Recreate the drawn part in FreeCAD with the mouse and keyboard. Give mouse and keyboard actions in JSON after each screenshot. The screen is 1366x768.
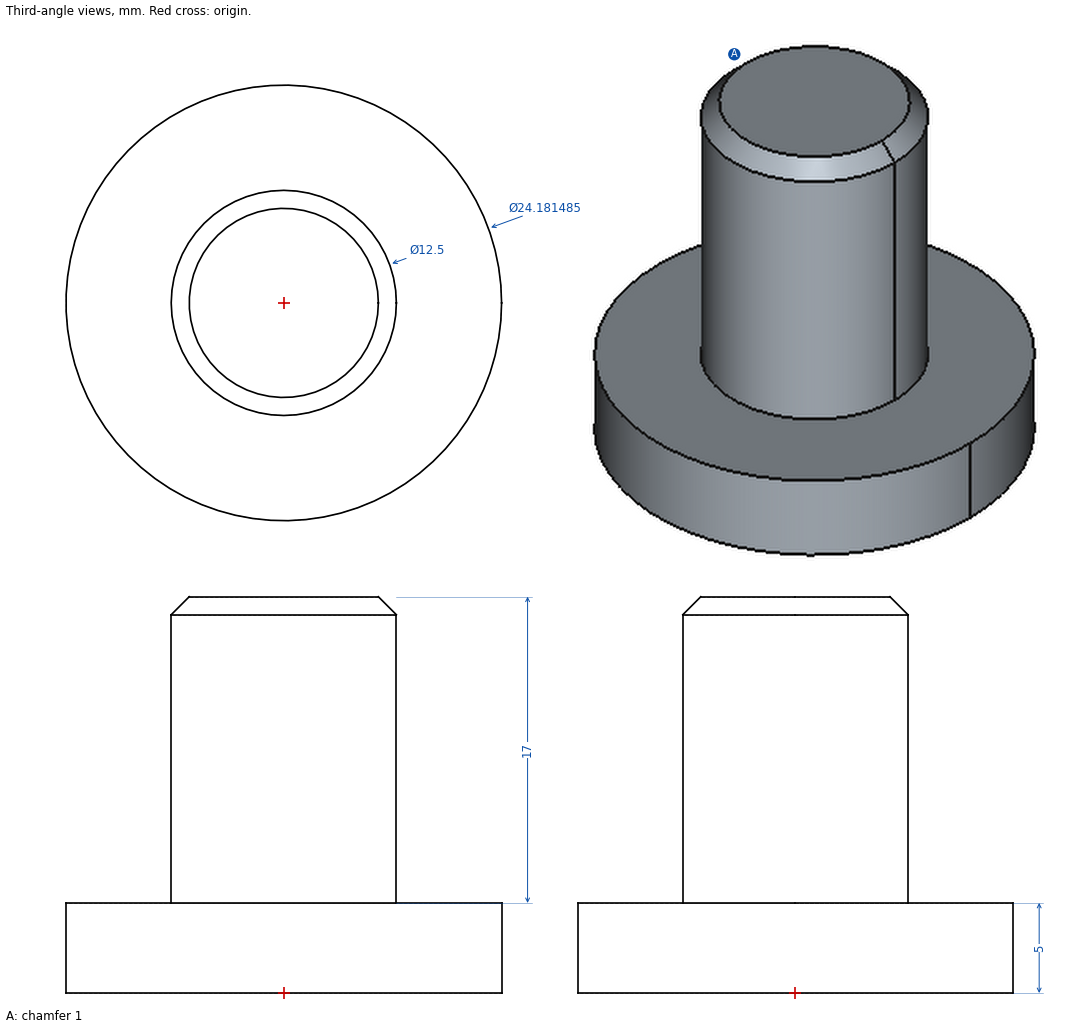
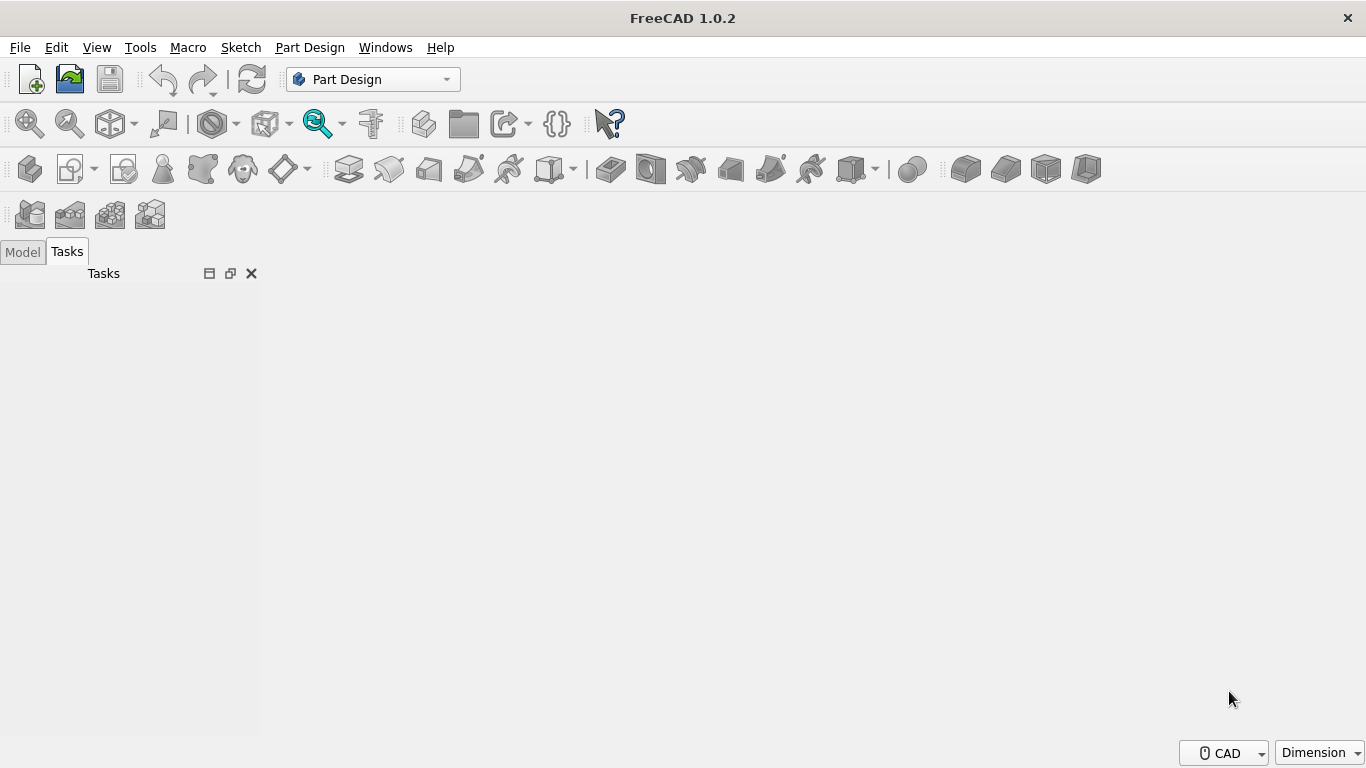
{"action": "left_click", "coordinate": [30, 80]}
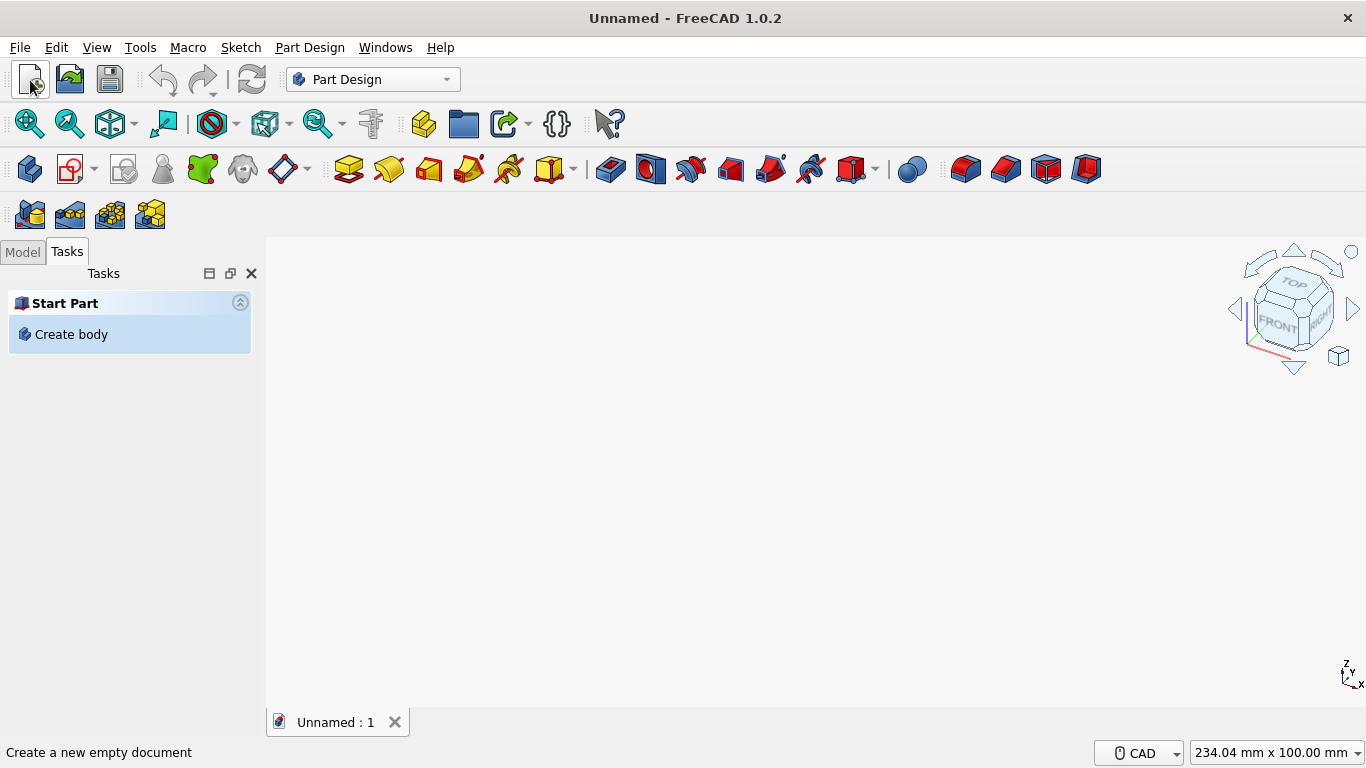
{"action": "left_click", "coordinate": [70, 170]}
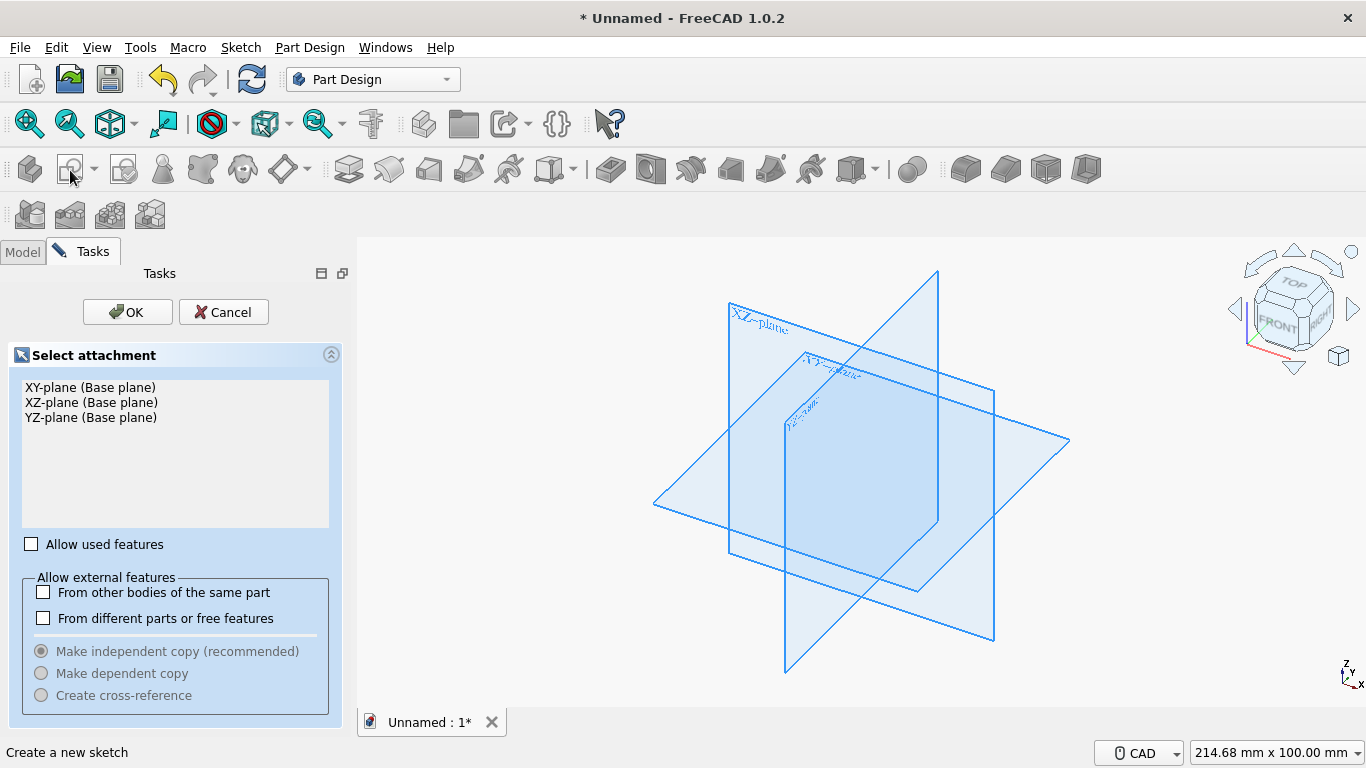
{"action": "left_click", "coordinate": [82, 388]}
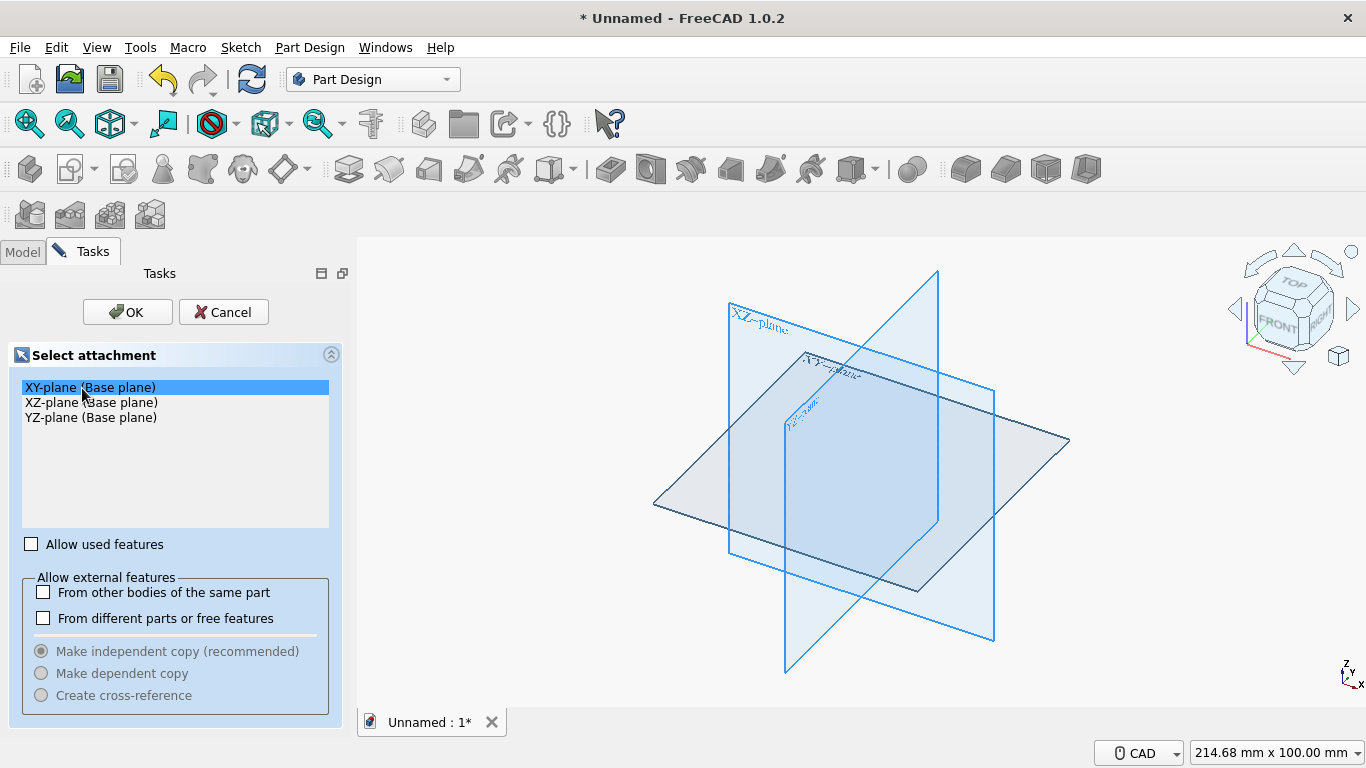
{"action": "left_click", "coordinate": [128, 312]}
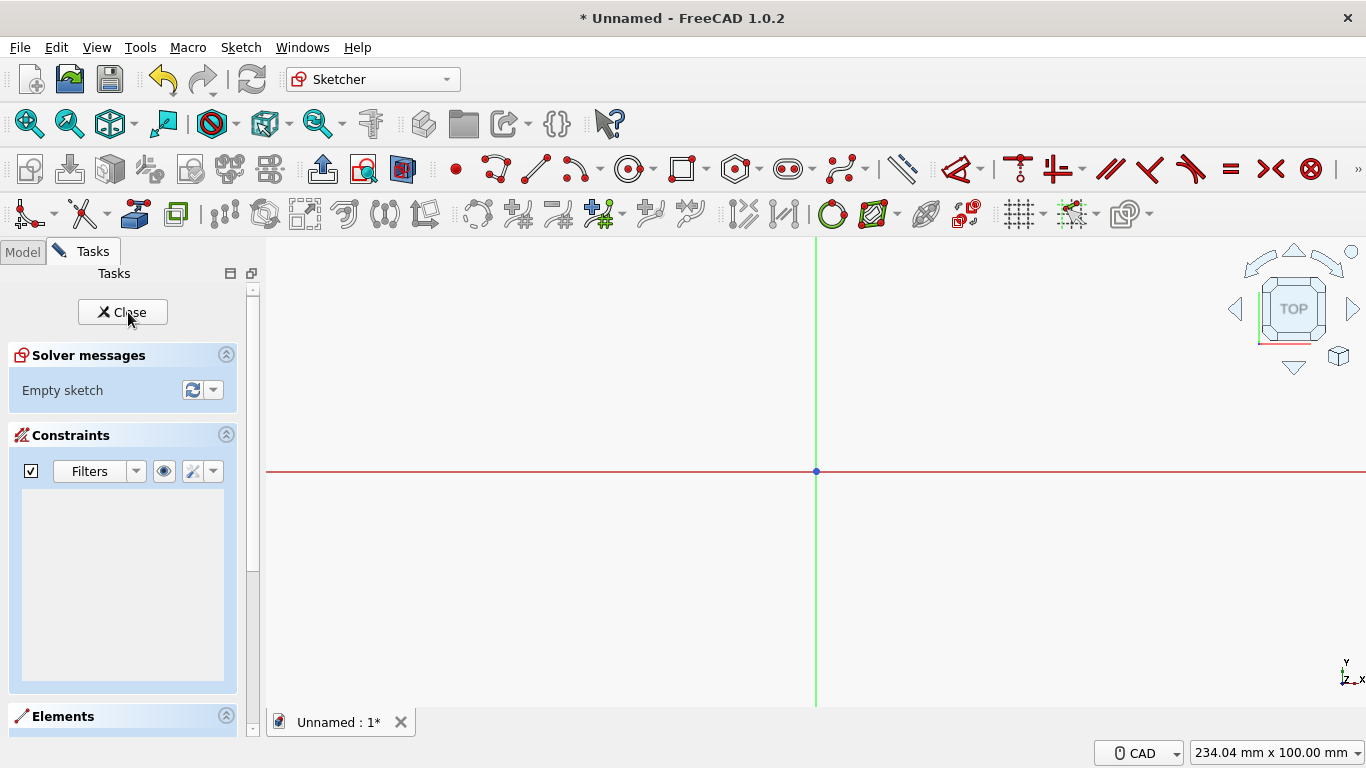
{"action": "scroll", "coordinate": [856, 472], "scroll_direction": "up", "scroll_amount": 5}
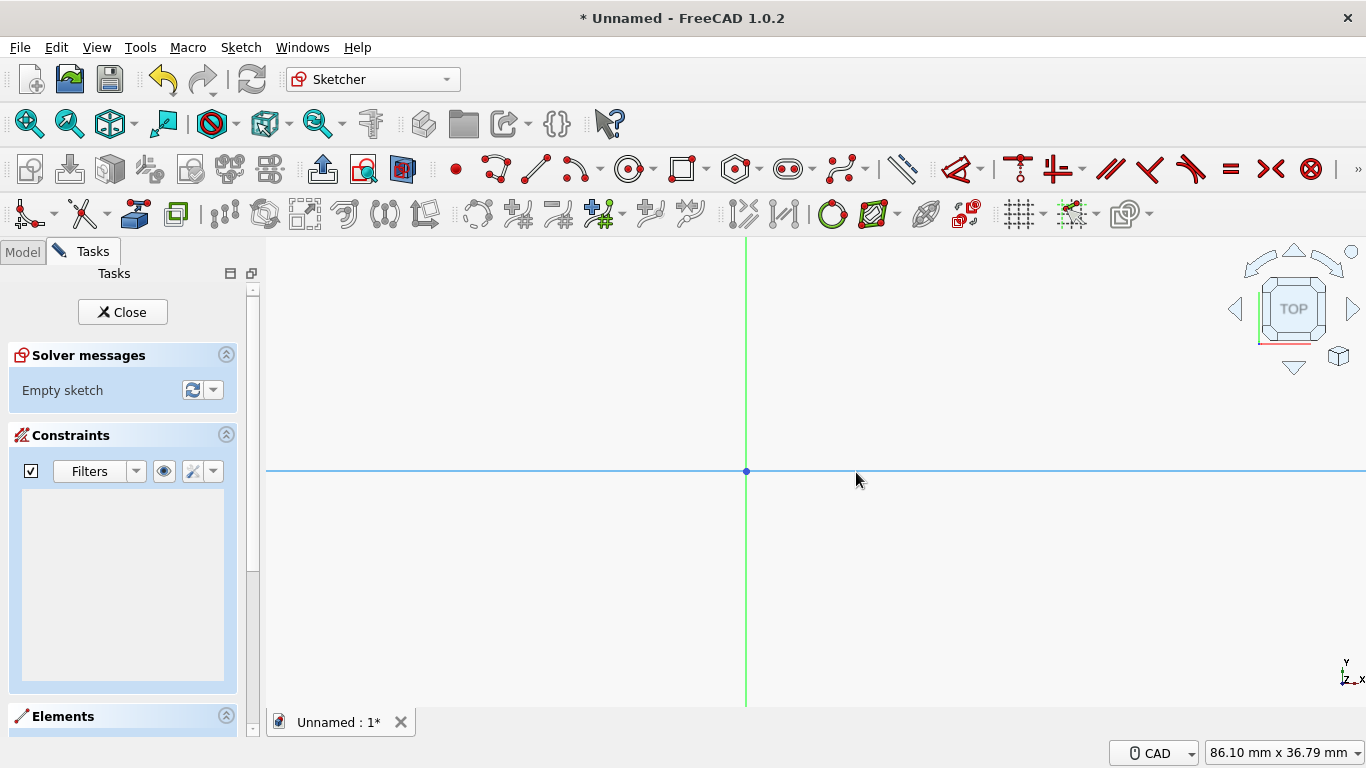
{"action": "left_click", "coordinate": [630, 170]}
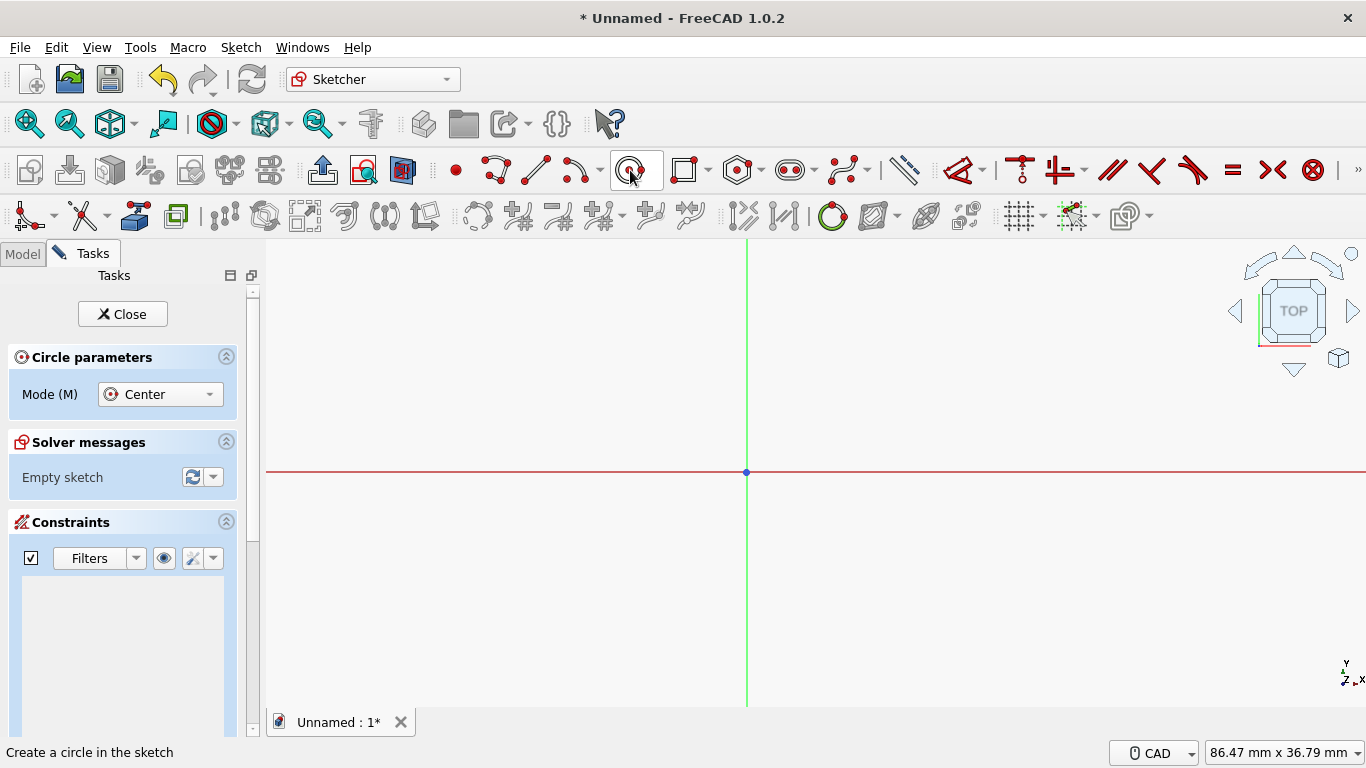
{"action": "left_click", "coordinate": [747, 472]}
{"action": "left_click", "coordinate": [855, 363]}
{"action": "key", "text": "Escape"}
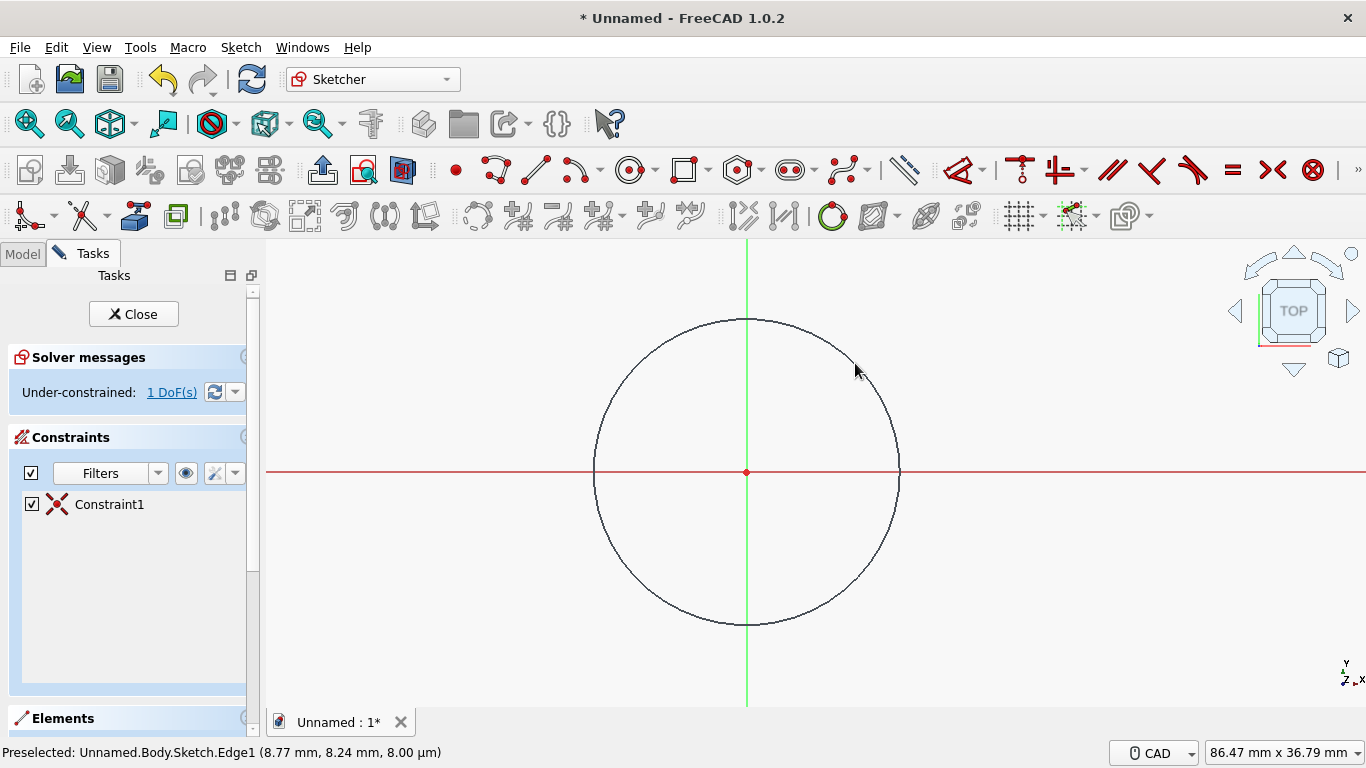
{"action": "left_click", "coordinate": [958, 170]}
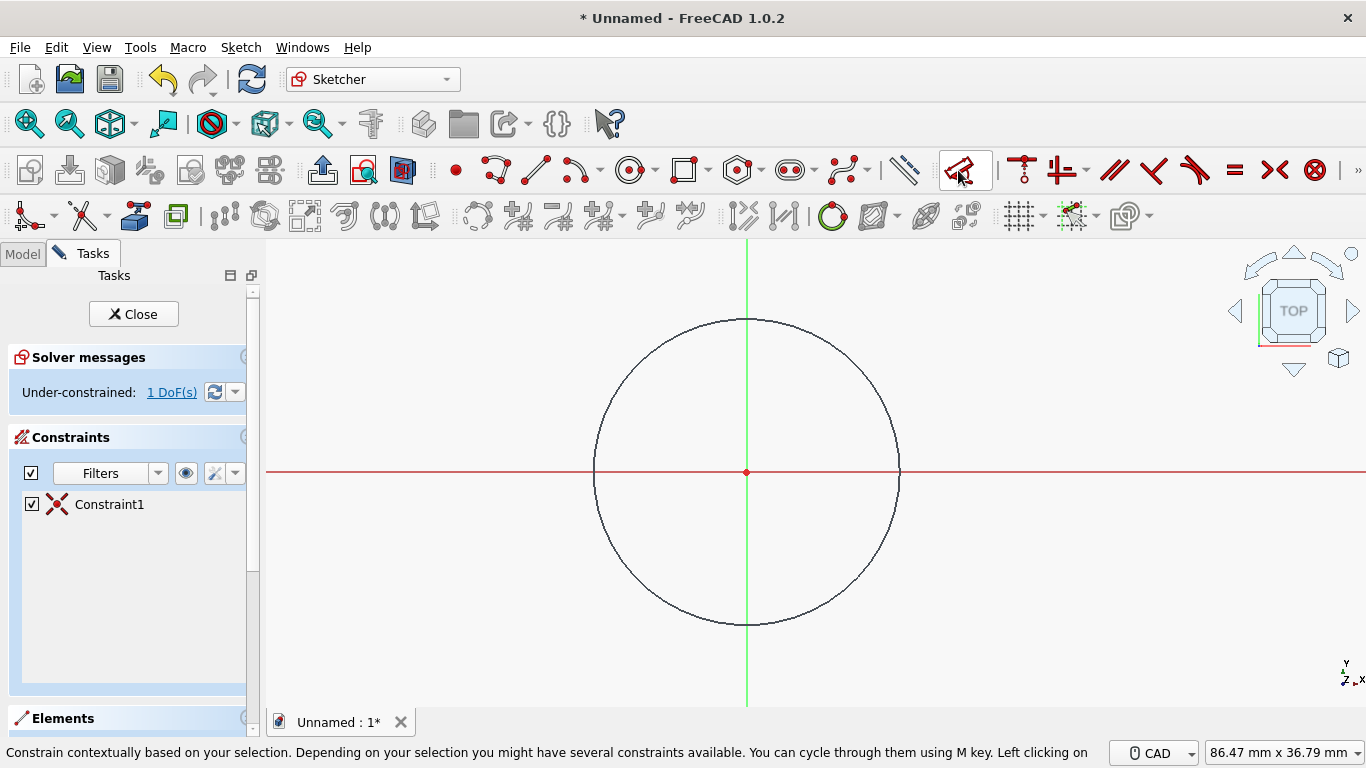
{"action": "left_click", "coordinate": [855, 364]}
{"action": "left_click", "coordinate": [878, 341]}